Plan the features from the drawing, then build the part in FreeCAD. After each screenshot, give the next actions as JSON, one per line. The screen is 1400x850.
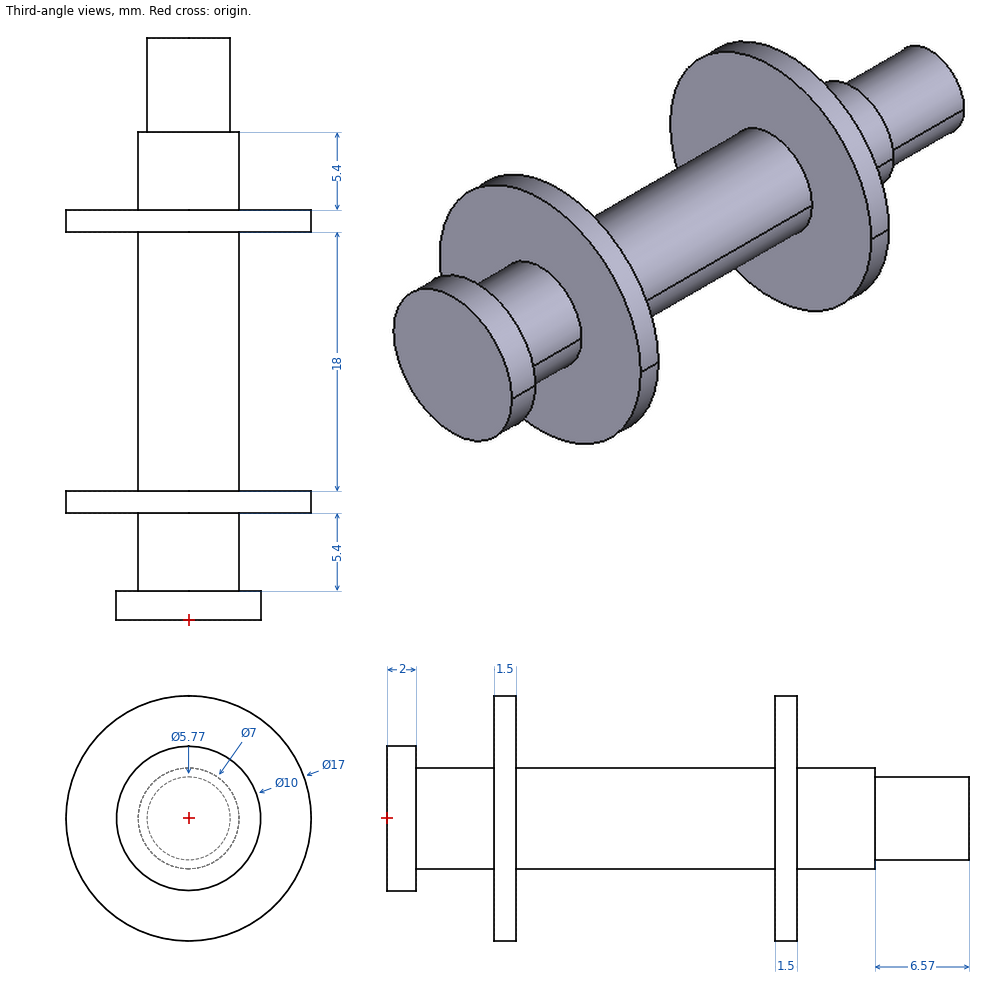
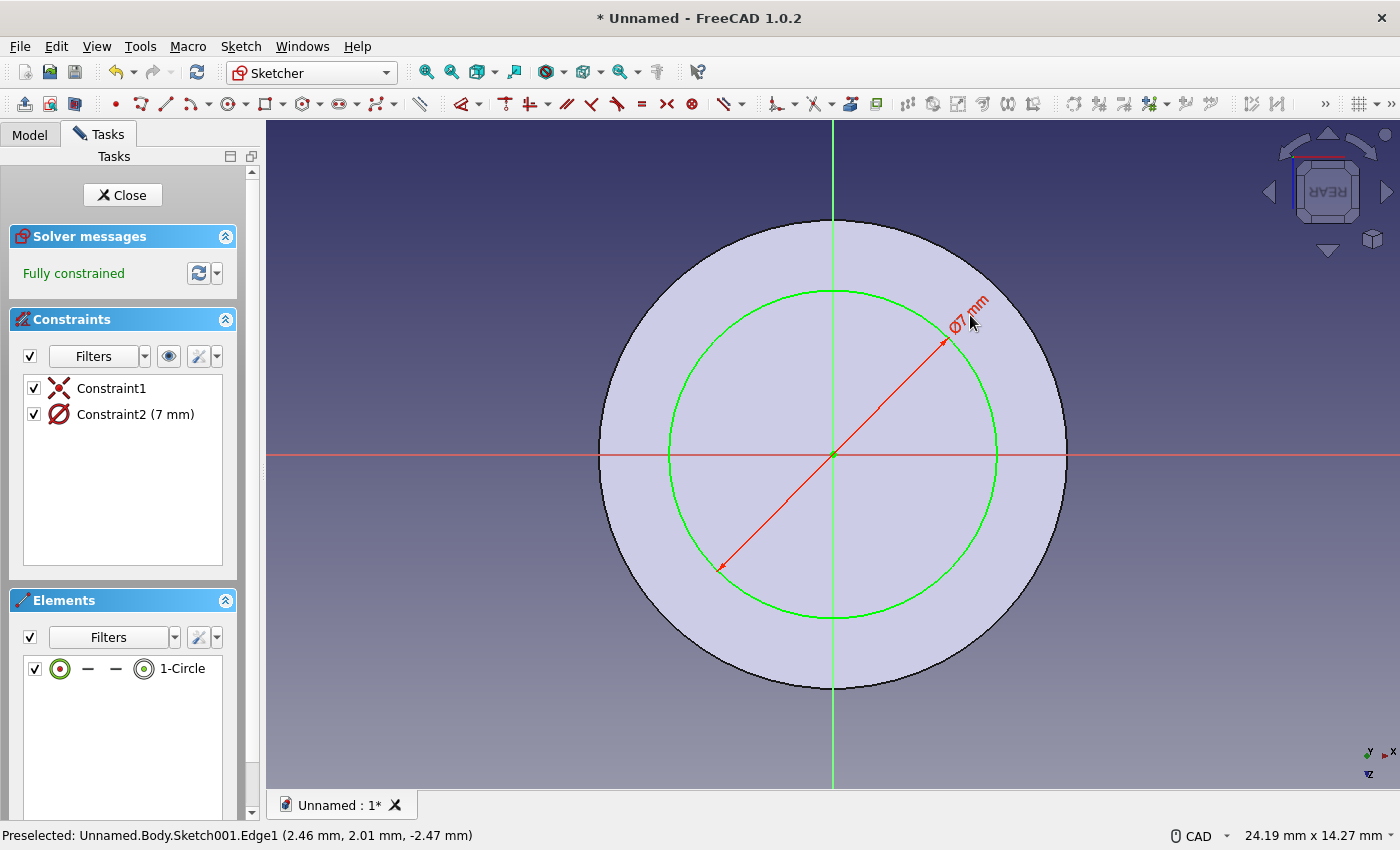
{"action": "left_click", "coordinate": [123, 195]}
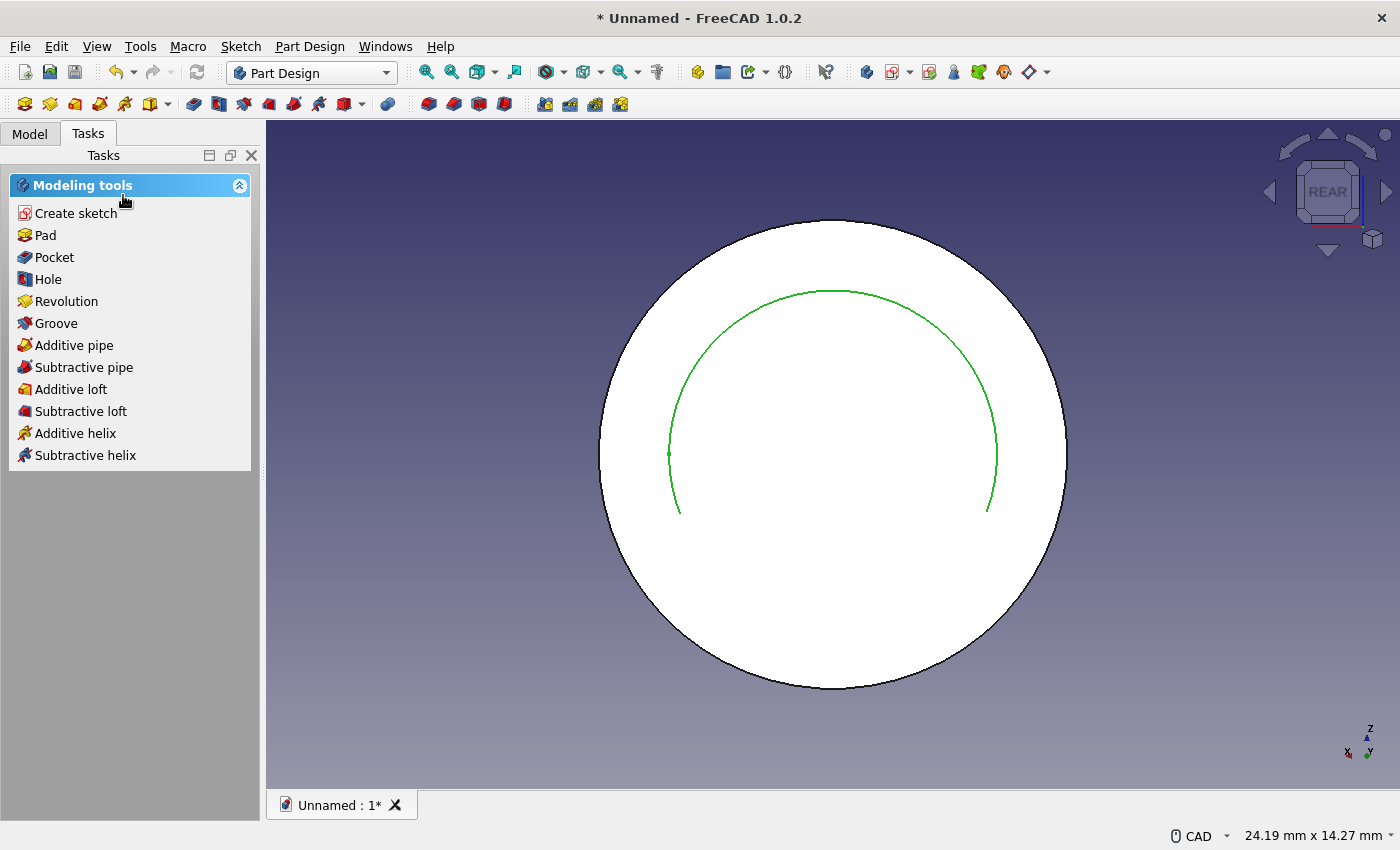
{"action": "left_click", "coordinate": [25, 104]}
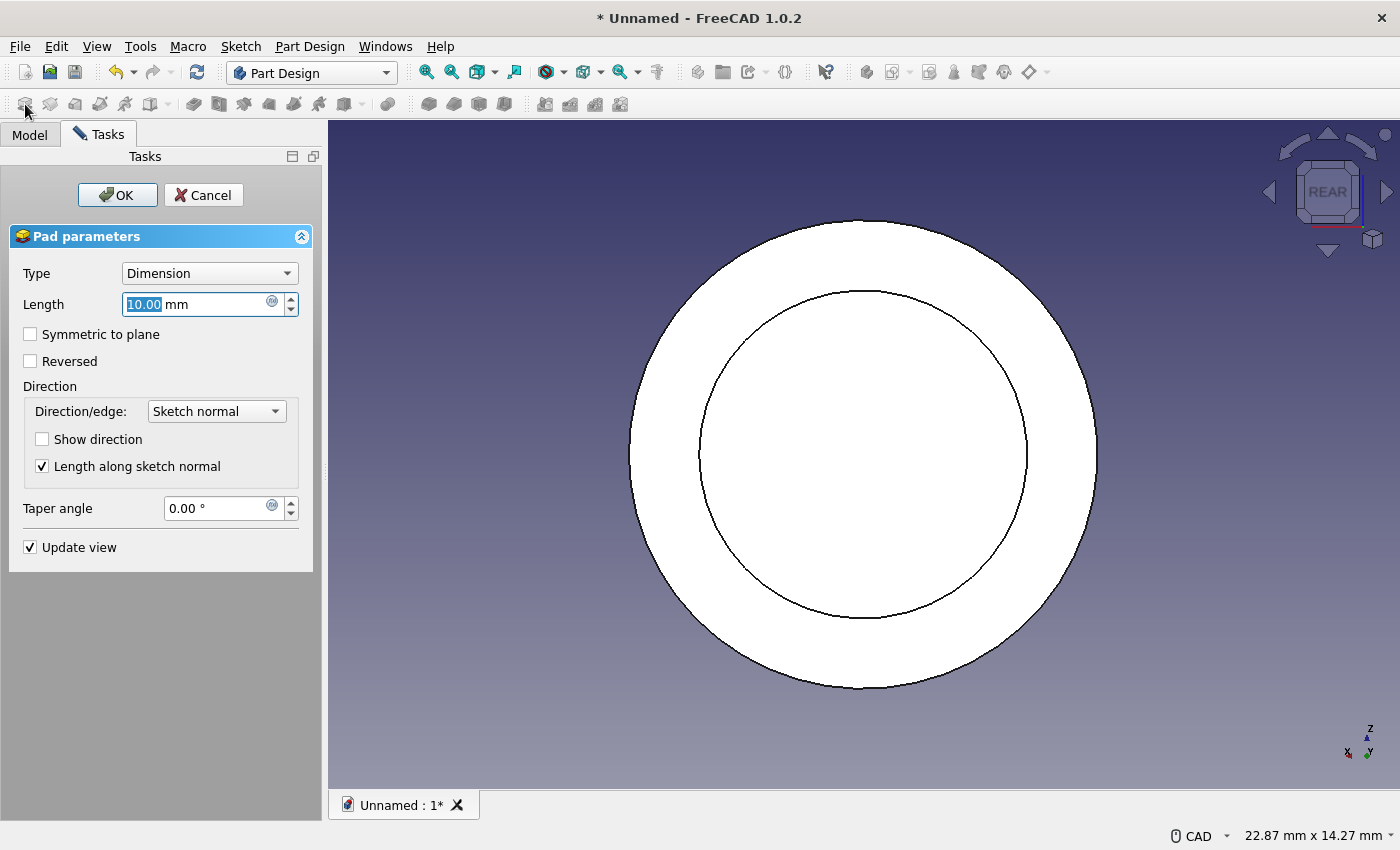
{"action": "type", "text": "5.4"}
{"action": "key", "text": "Tab"}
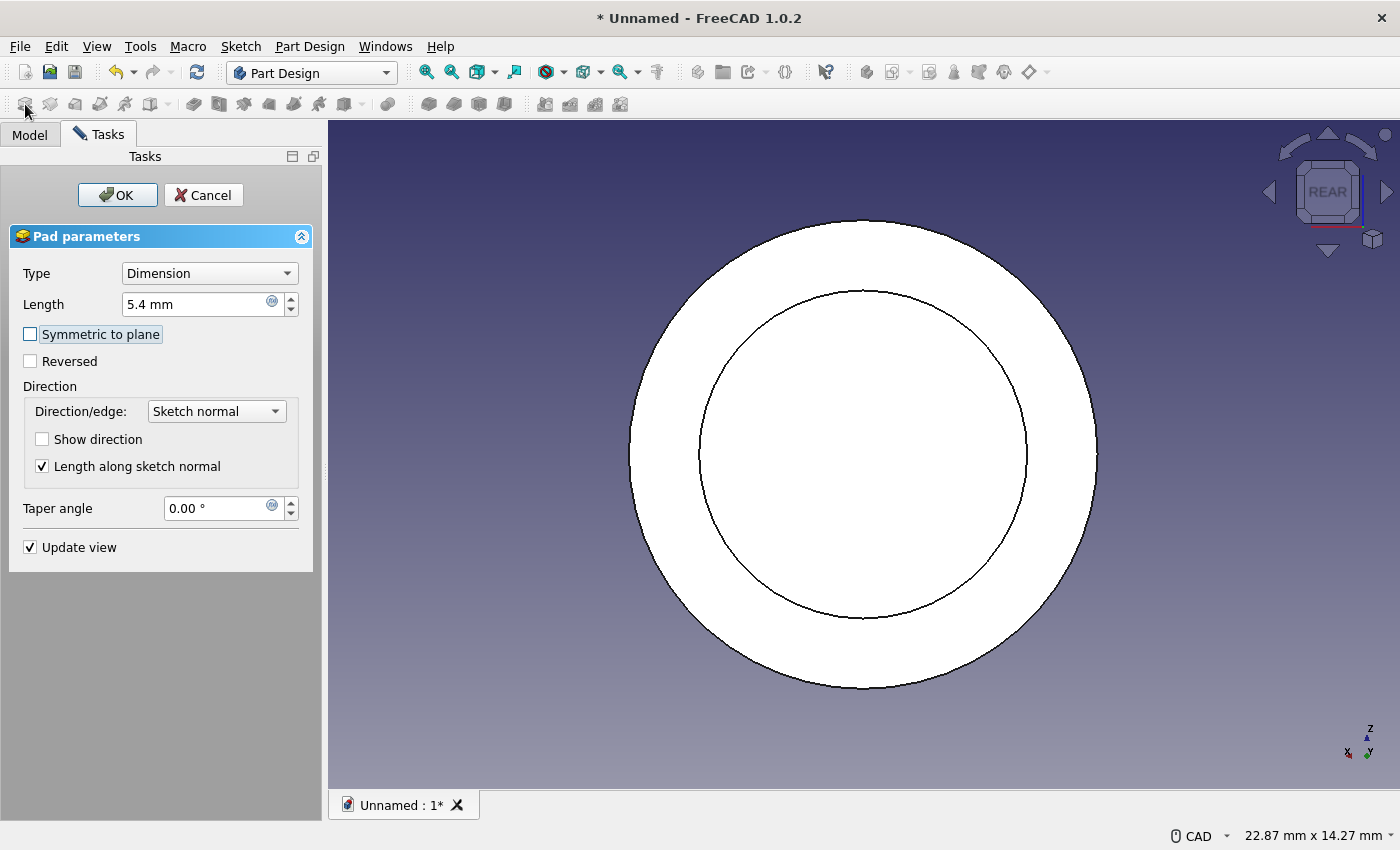
{"action": "left_click", "coordinate": [118, 195]}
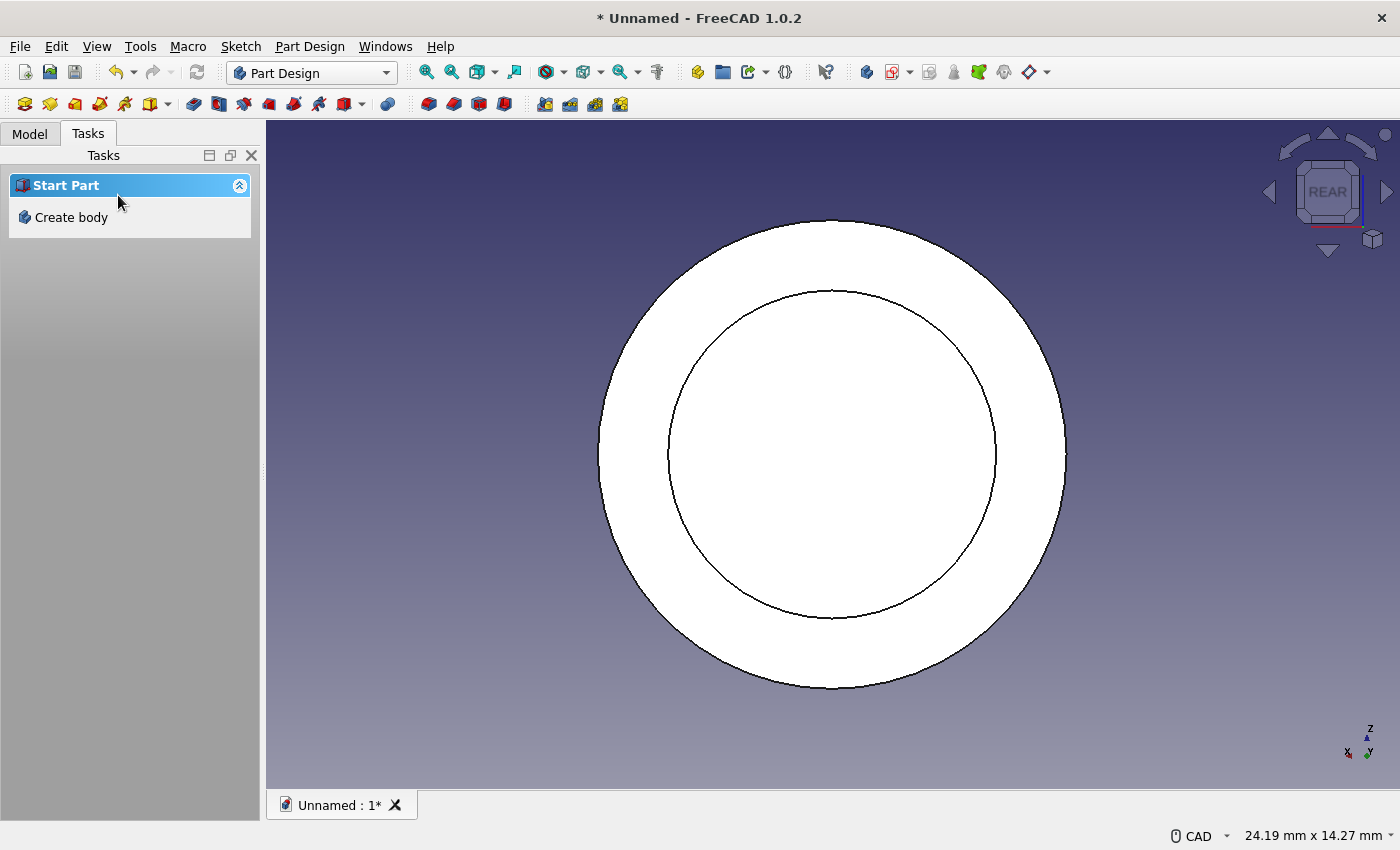
{"action": "left_click", "coordinate": [832, 454]}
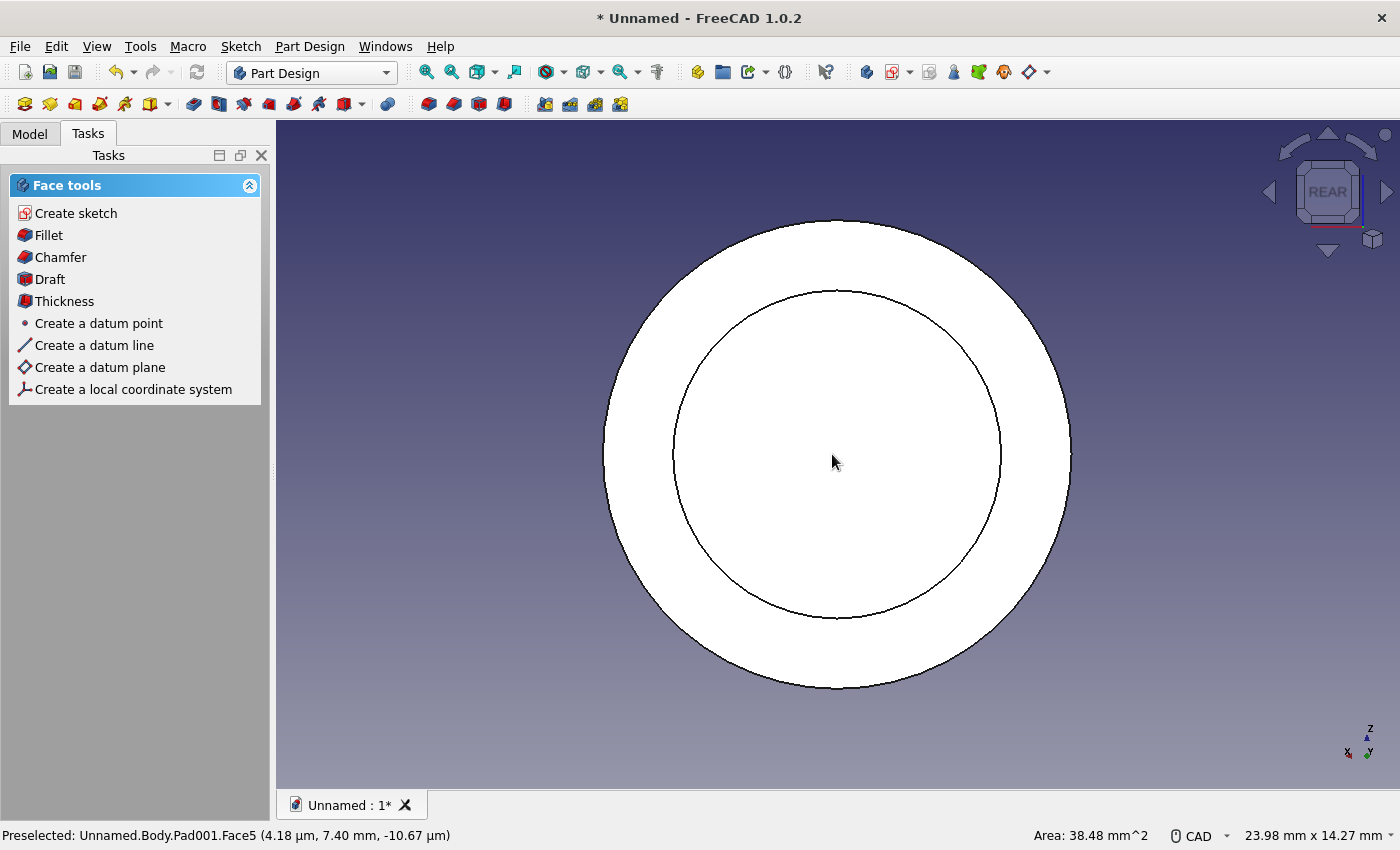
{"action": "left_click", "coordinate": [892, 72]}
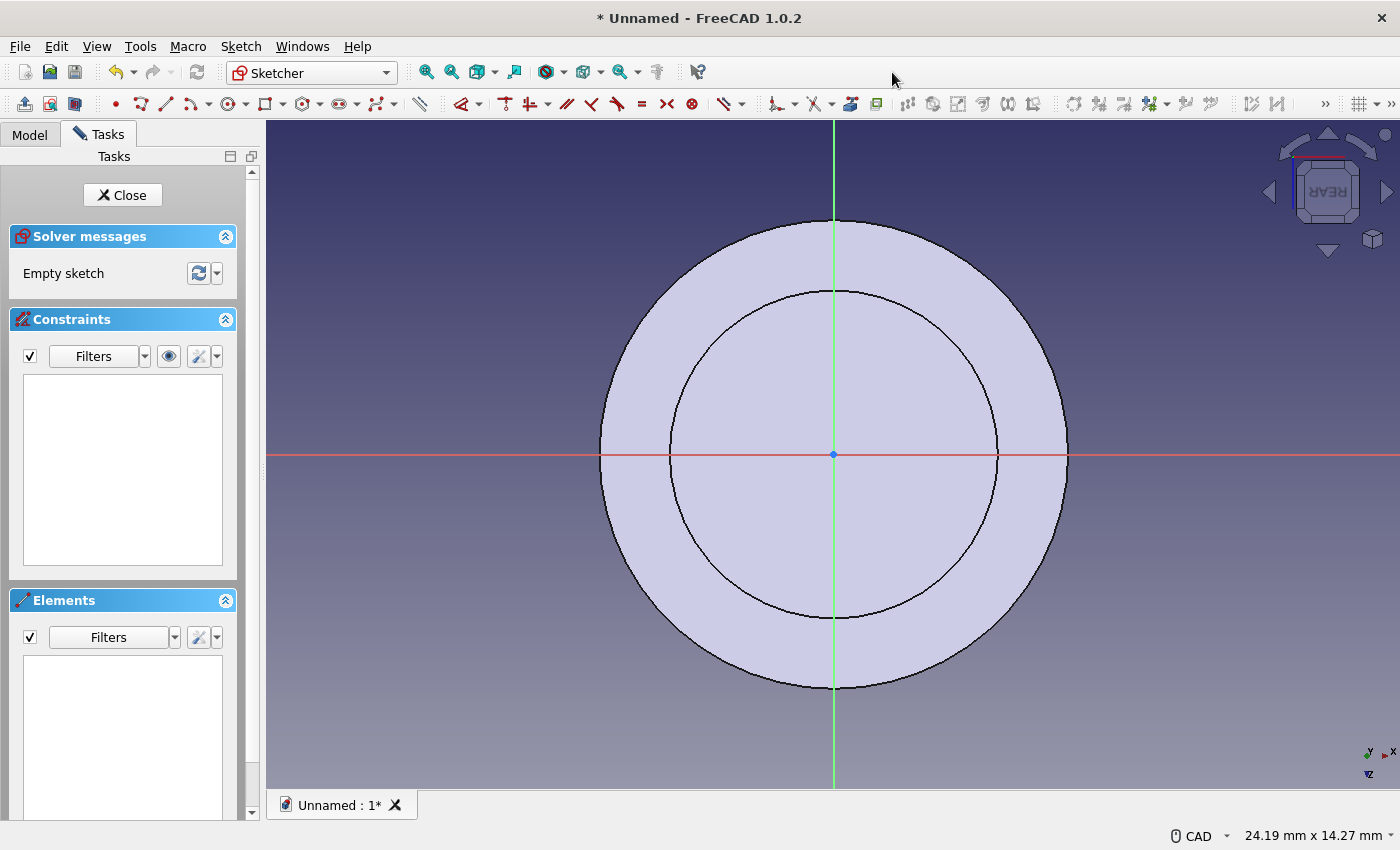
{"action": "scroll", "coordinate": [680, 455], "scroll_direction": "down", "scroll_amount": 3}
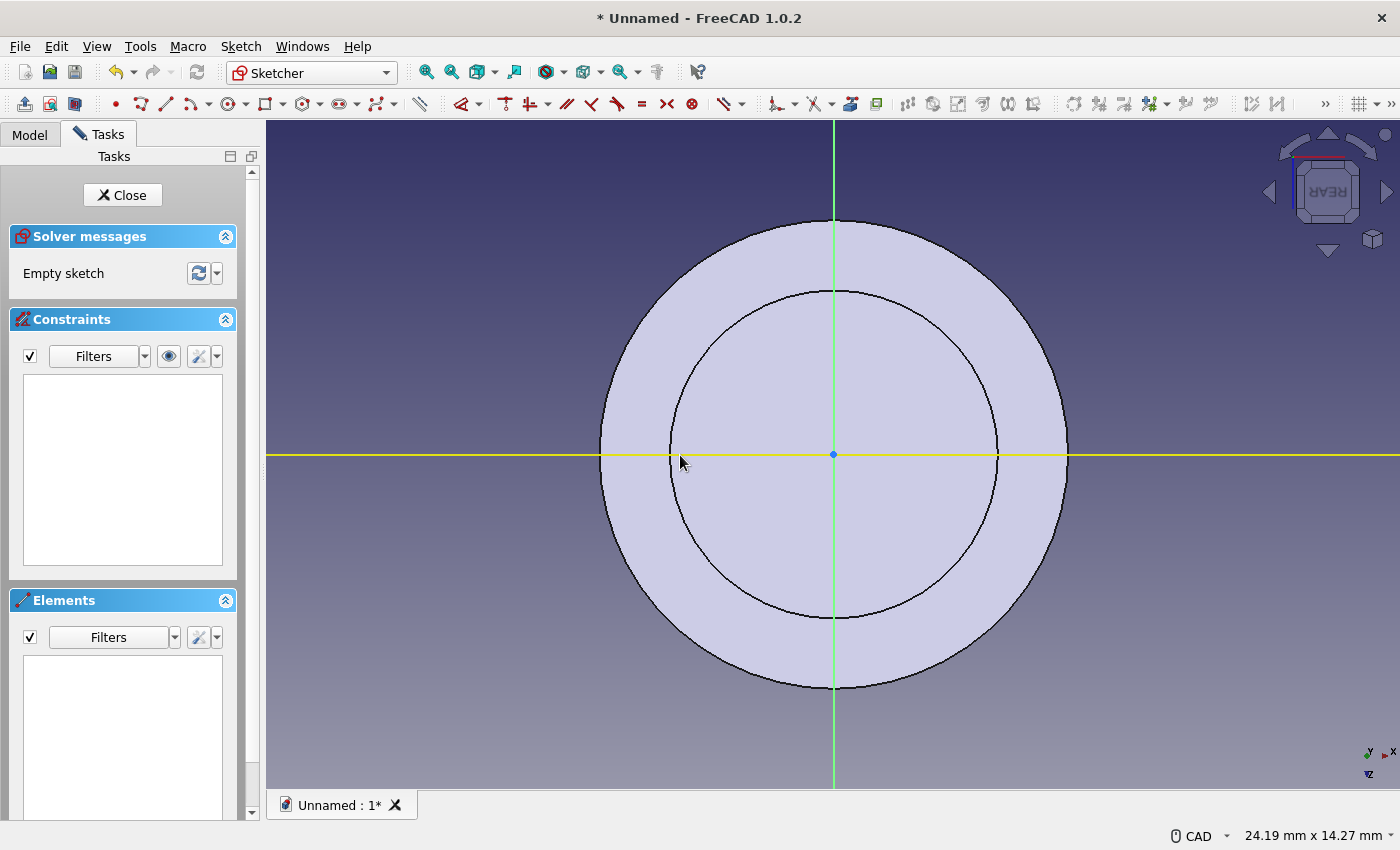
{"action": "left_click", "coordinate": [228, 104]}